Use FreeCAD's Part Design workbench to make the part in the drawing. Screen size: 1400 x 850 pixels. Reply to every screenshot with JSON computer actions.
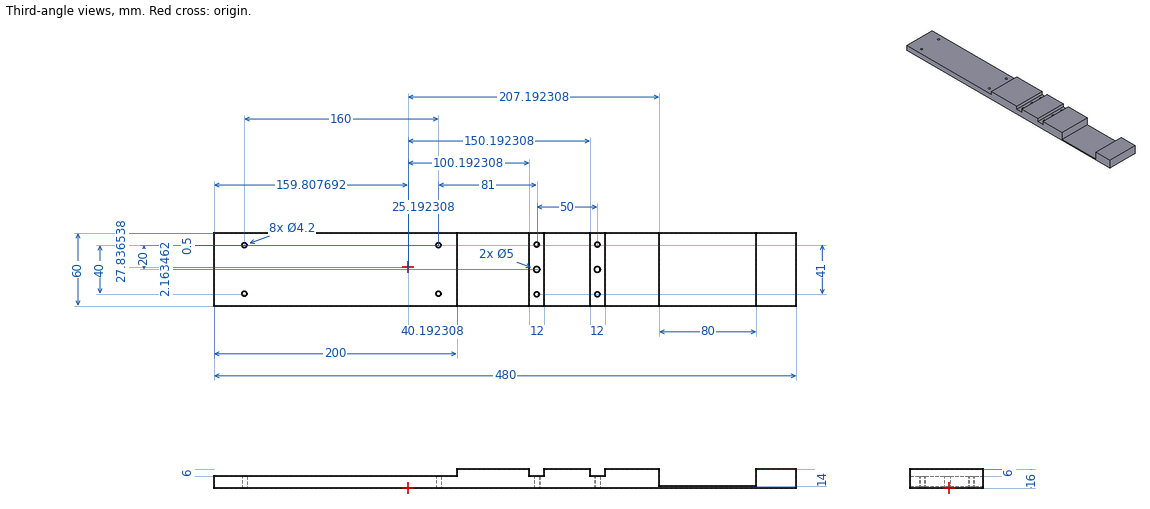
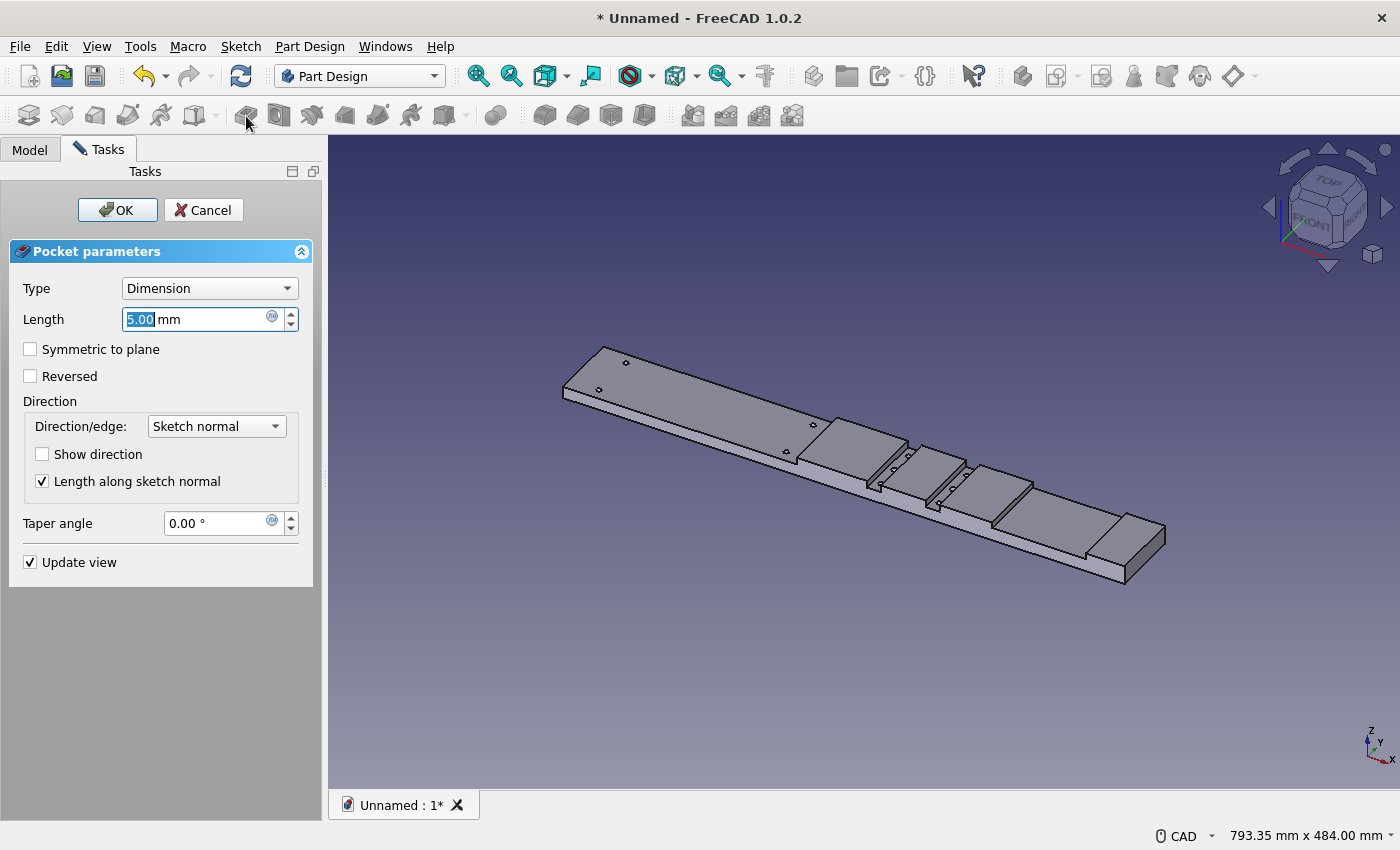
{"action": "type", "text": "14"}
{"action": "key", "text": "Tab"}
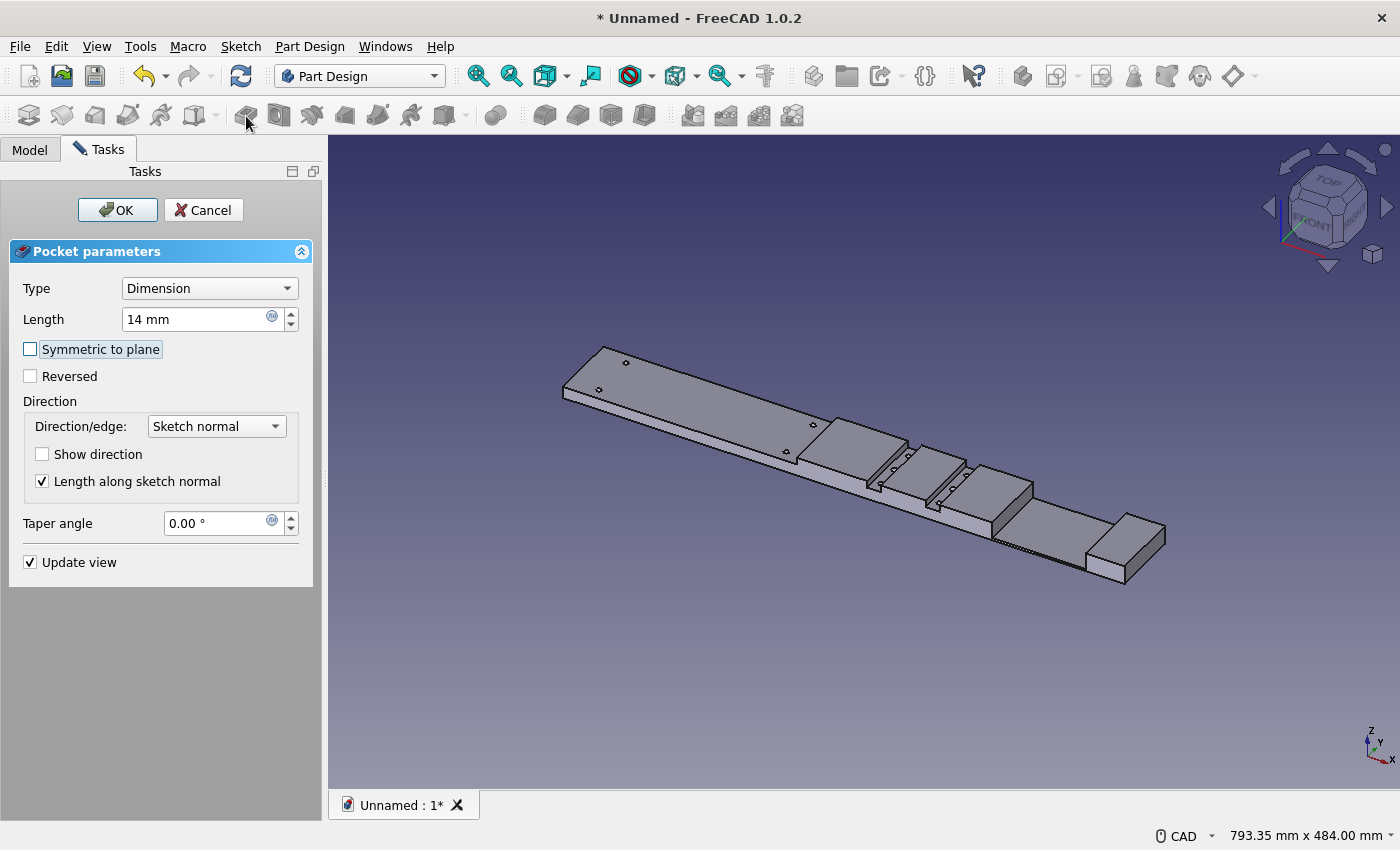
{"action": "left_click", "coordinate": [118, 210]}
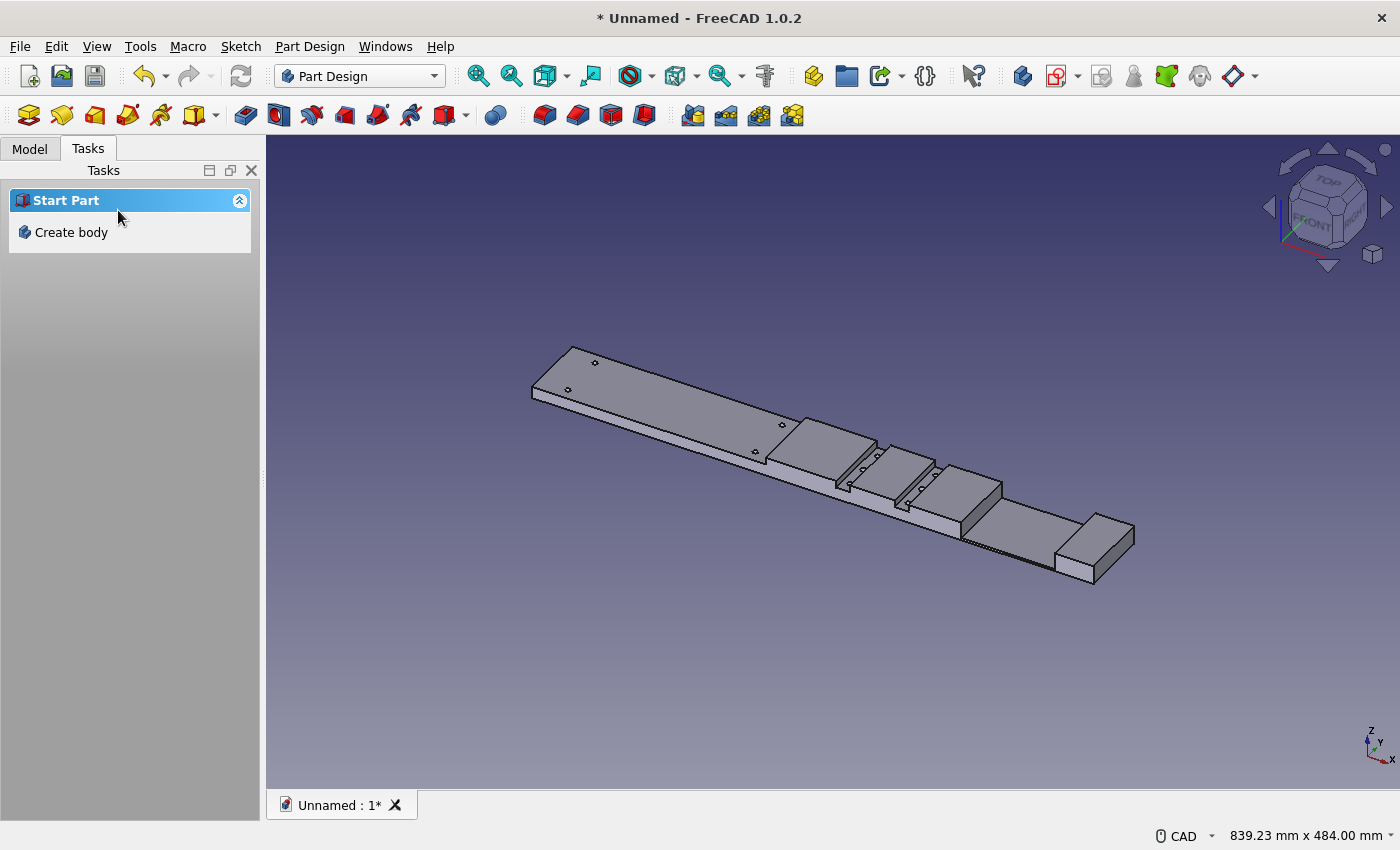
{"action": "key", "text": "0"}